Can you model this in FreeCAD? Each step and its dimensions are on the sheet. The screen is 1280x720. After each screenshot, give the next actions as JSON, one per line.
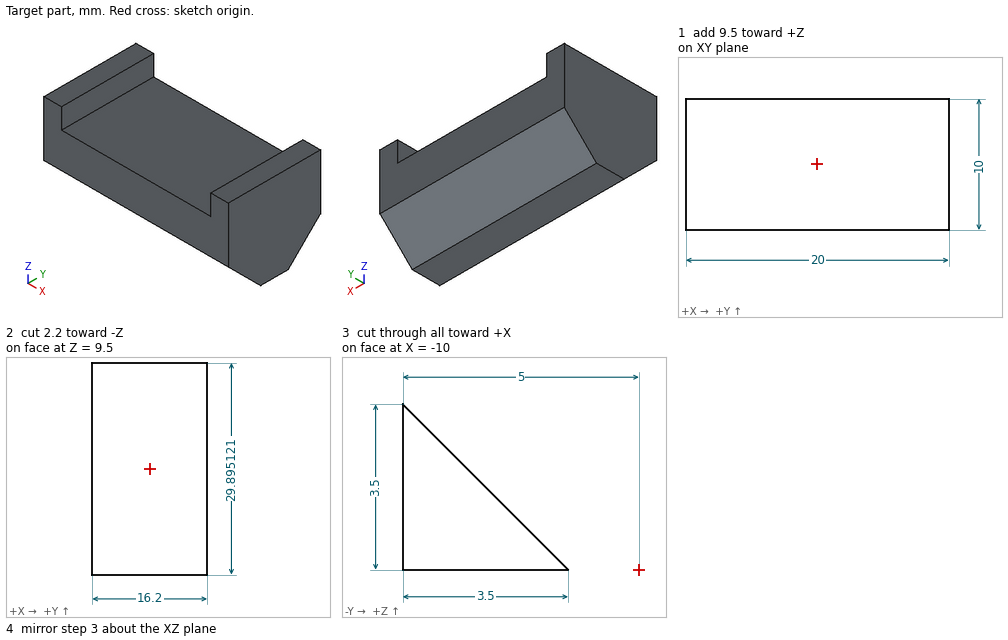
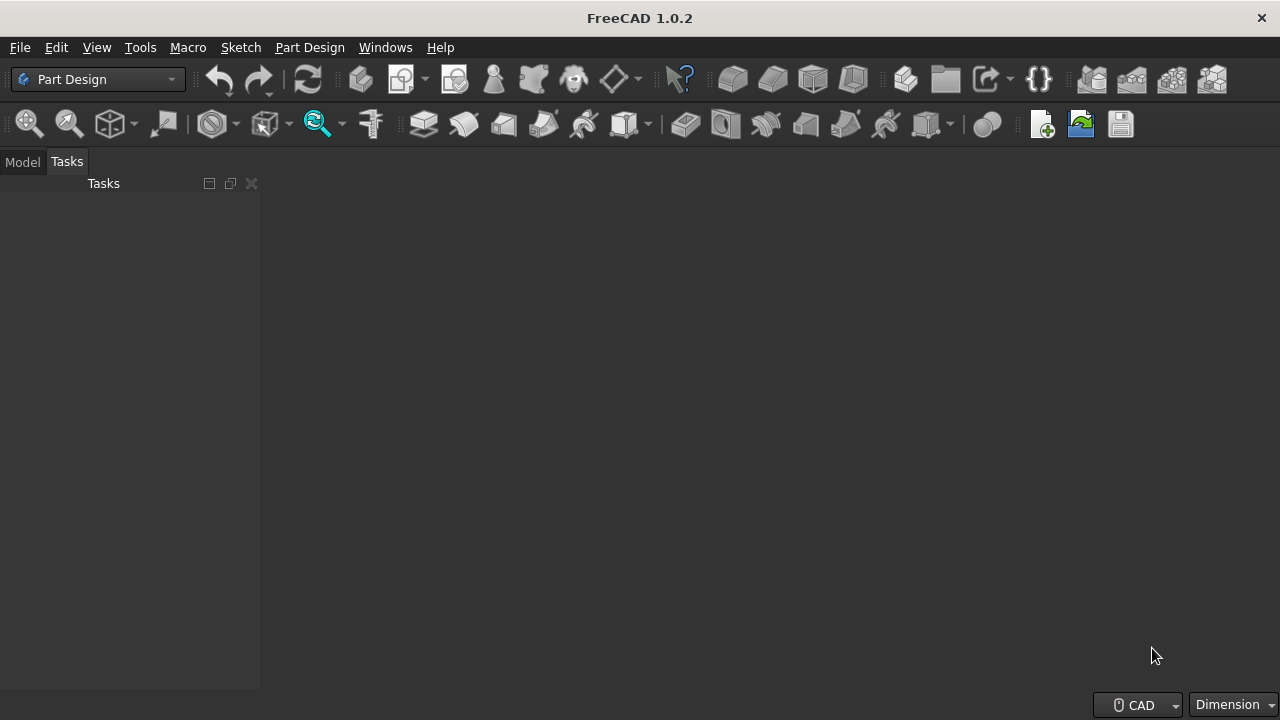
{"action": "left_click", "coordinate": [1042, 124]}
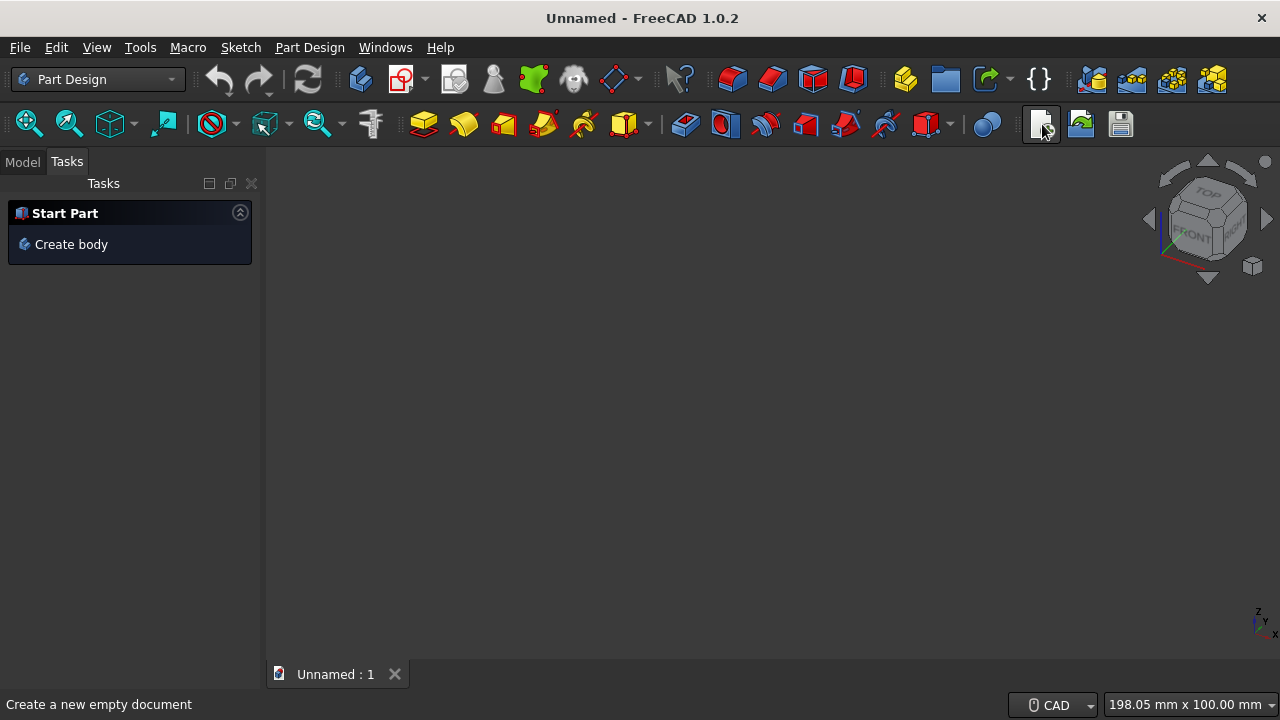
{"action": "left_click", "coordinate": [402, 80]}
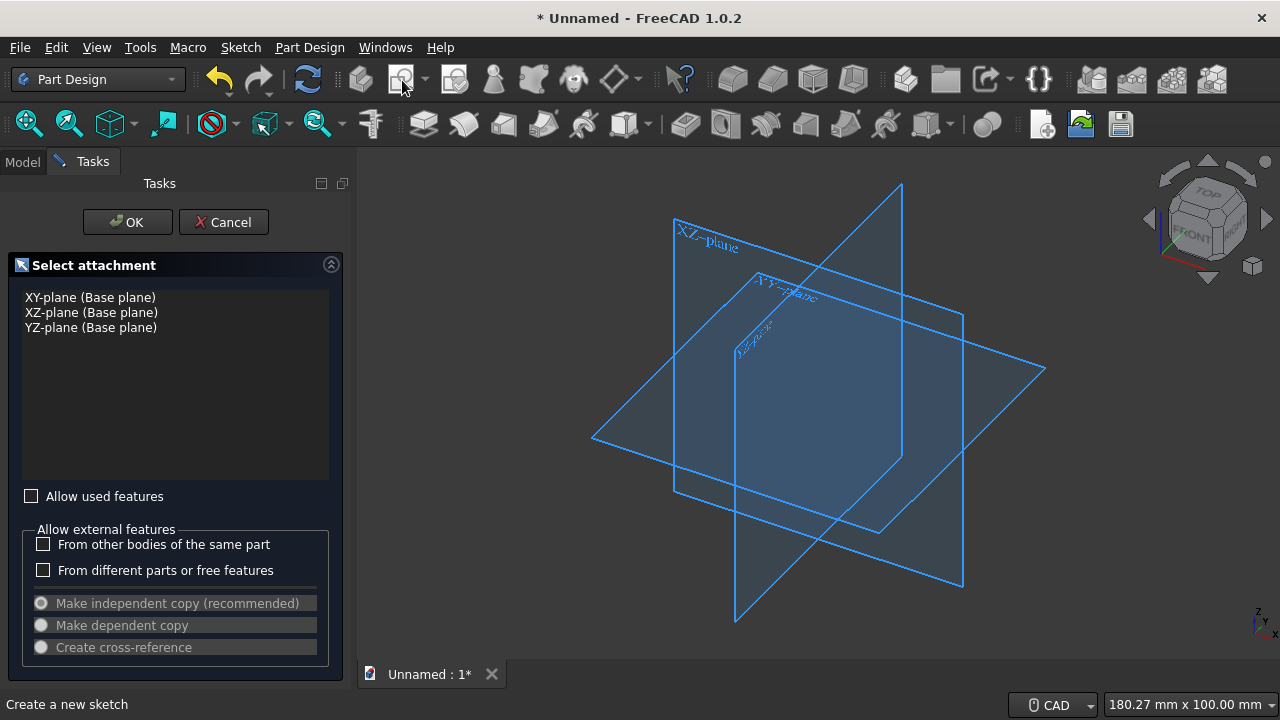
{"action": "left_click", "coordinate": [82, 298]}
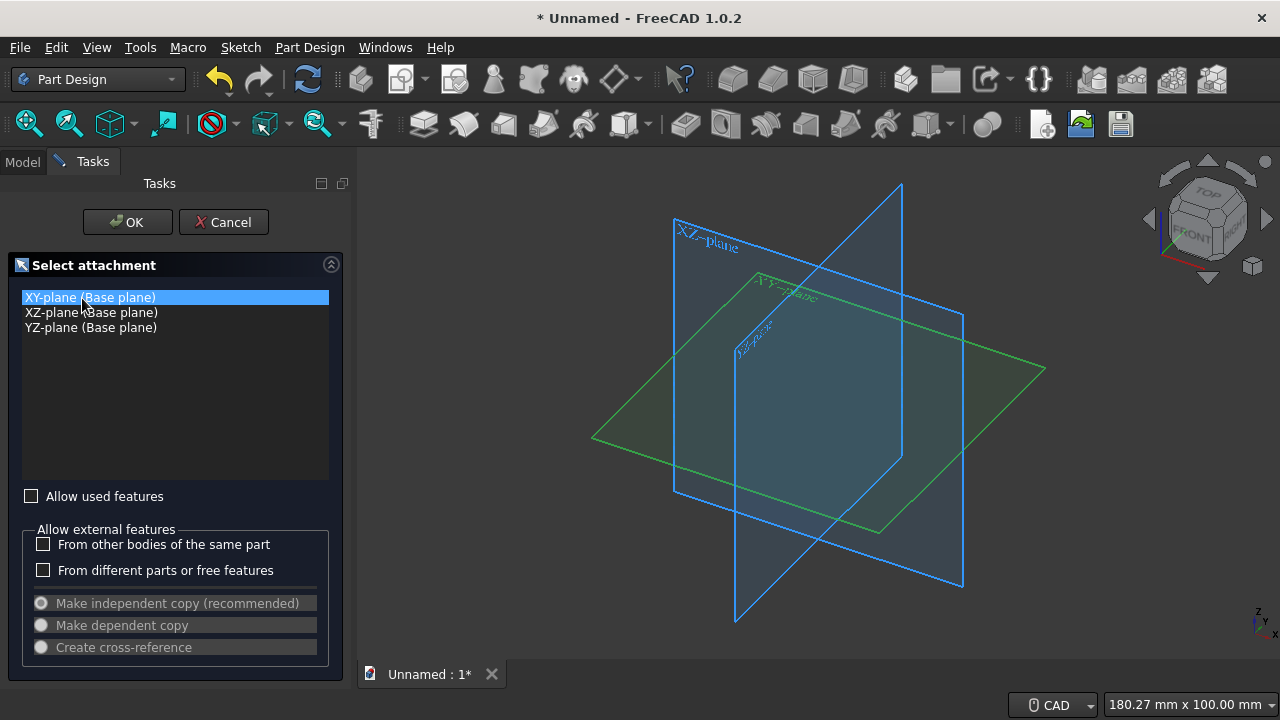
{"action": "left_click", "coordinate": [128, 222]}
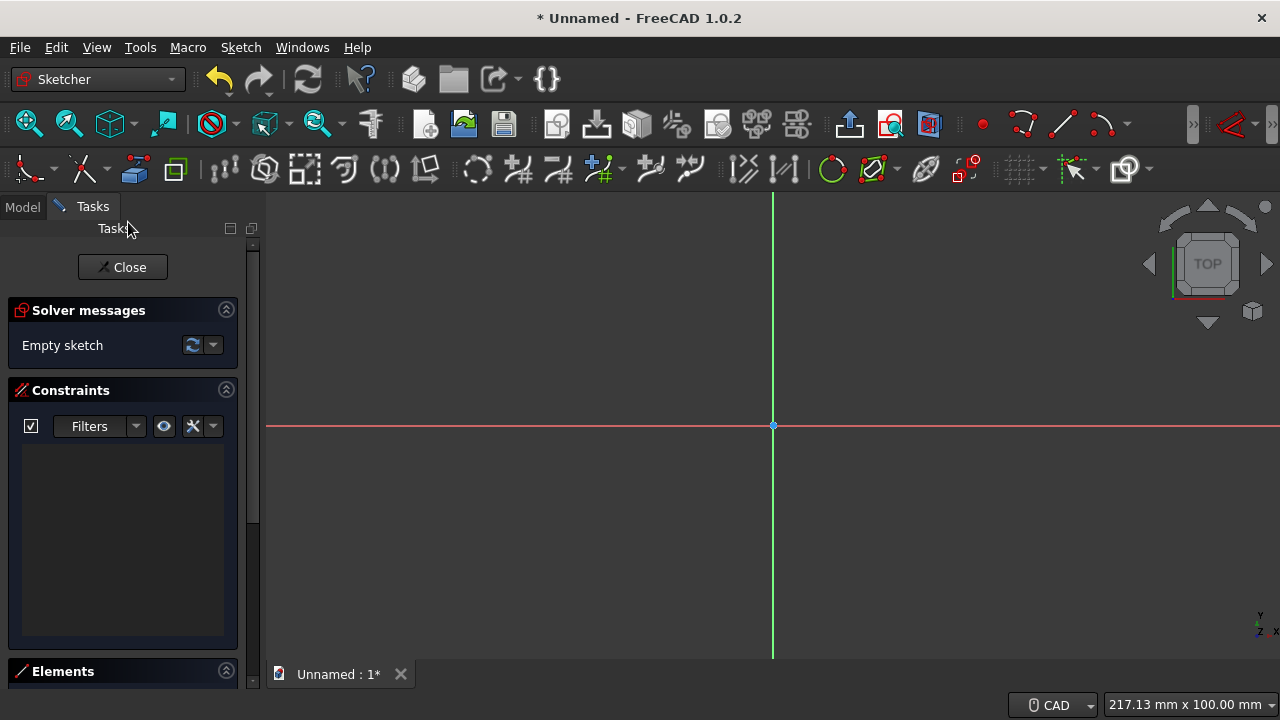
{"action": "scroll", "coordinate": [787, 426], "scroll_direction": "up", "scroll_amount": 9}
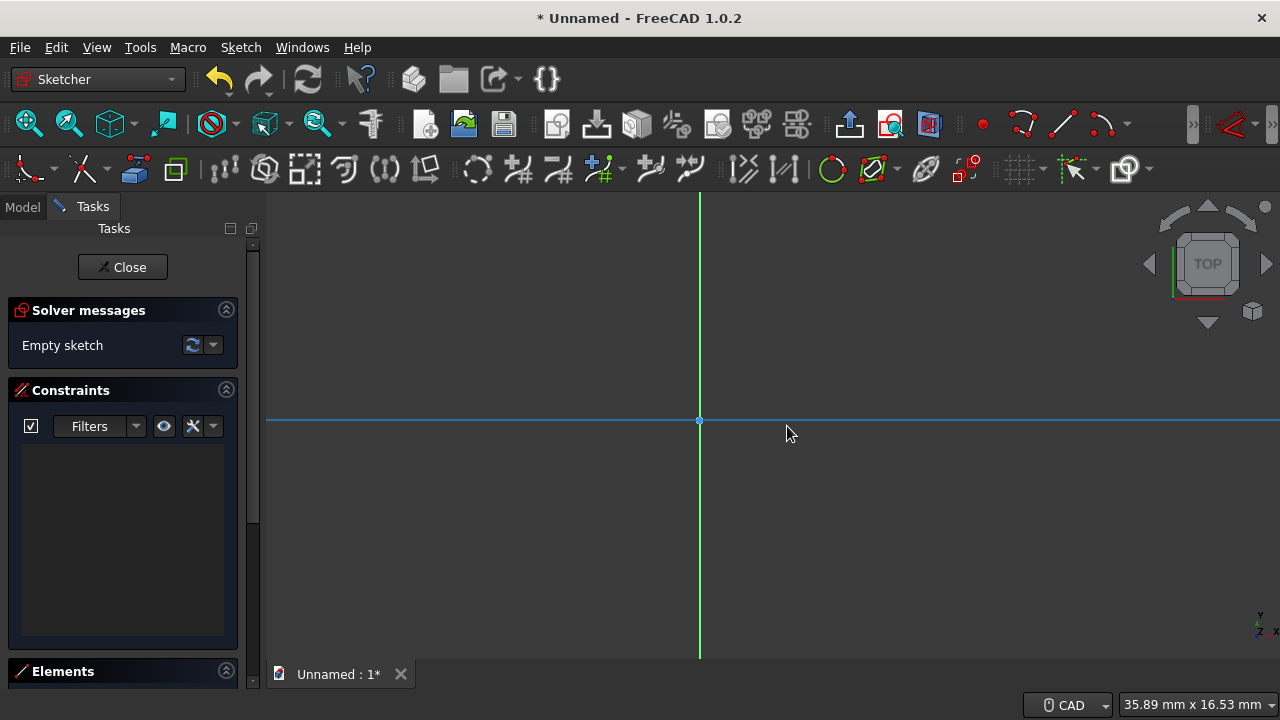
{"action": "key", "text": "g v"}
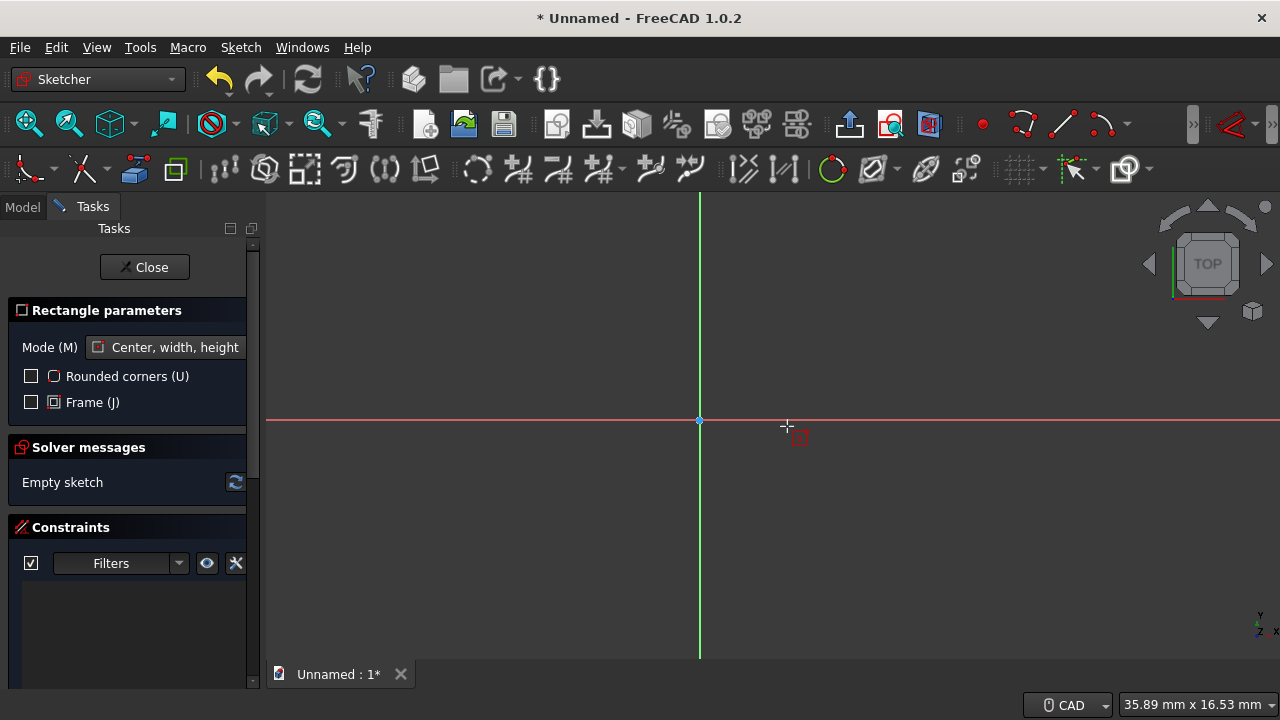
{"action": "left_click", "coordinate": [700, 420]}
{"action": "left_click", "coordinate": [982, 279]}
{"action": "key", "text": "Escape"}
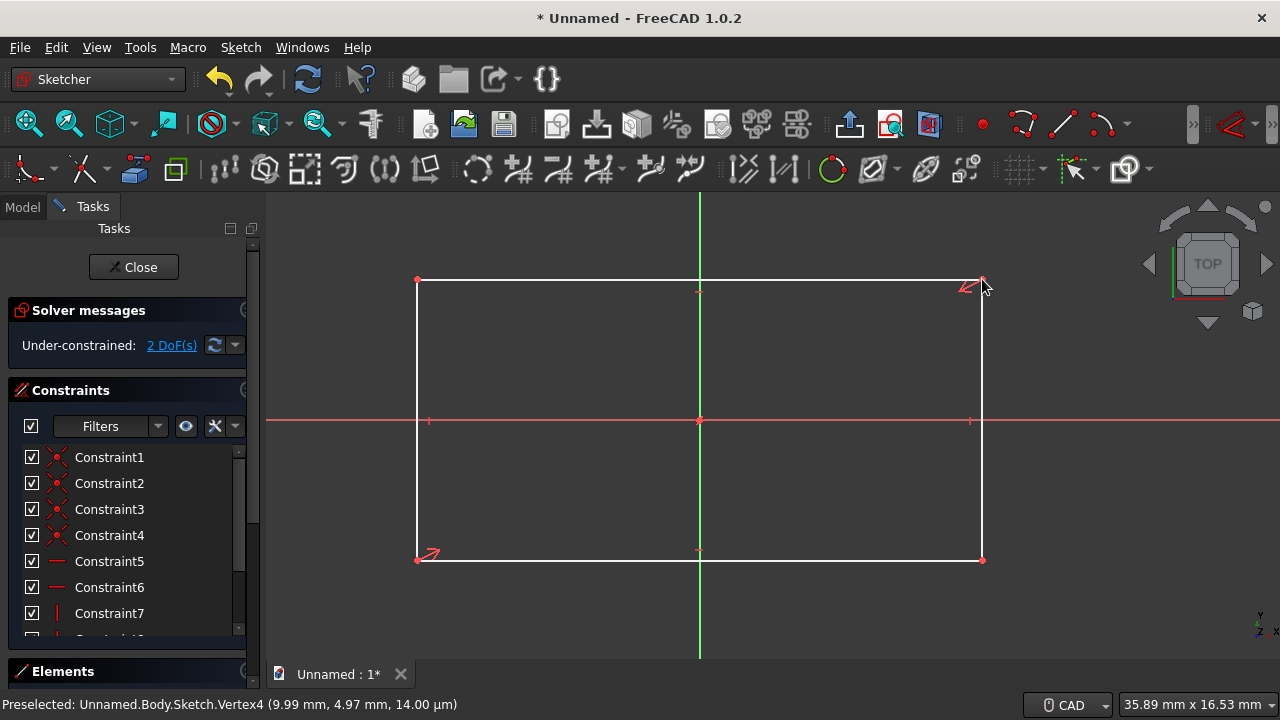
{"action": "left_click", "coordinate": [587, 561]}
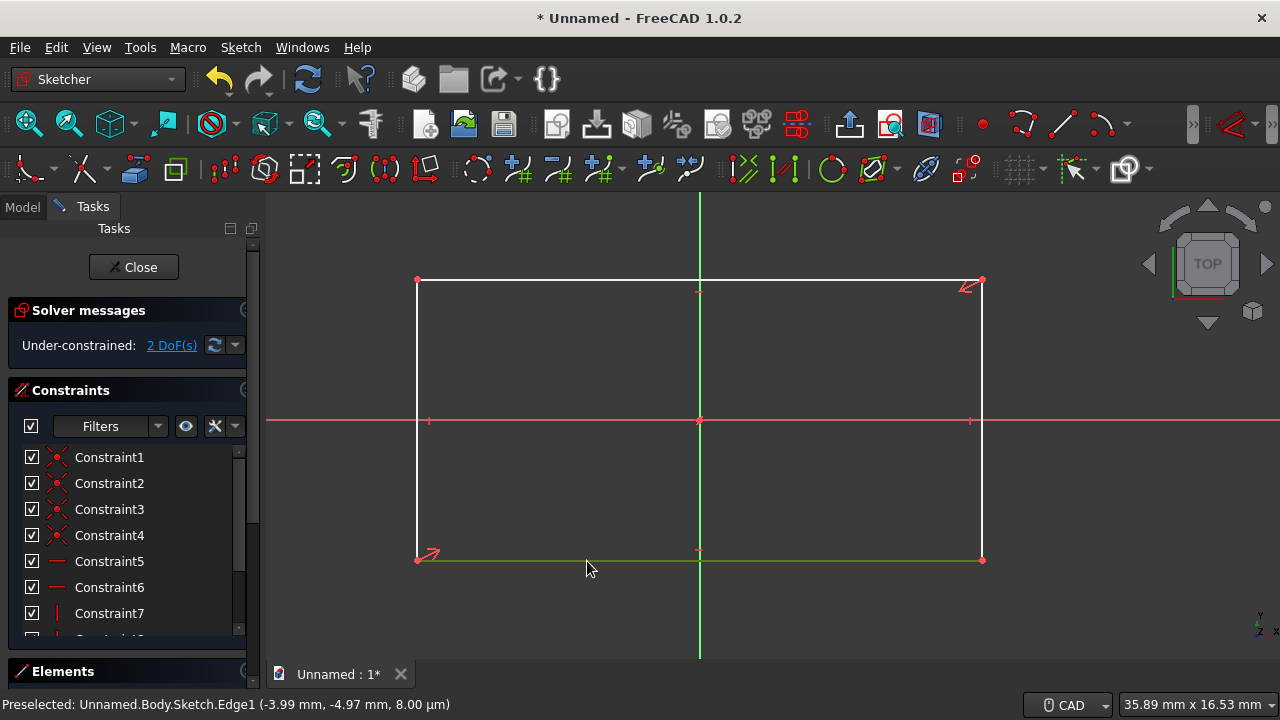
{"action": "left_click", "coordinate": [1258, 124]}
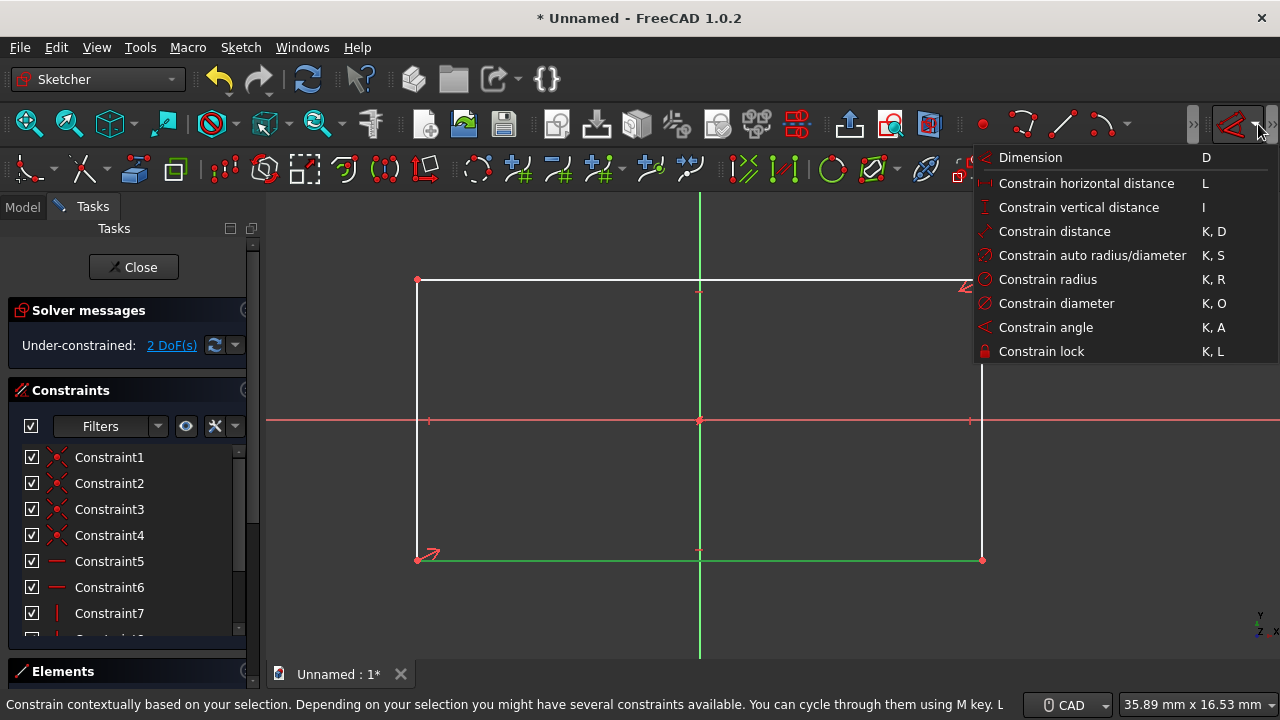
{"action": "left_click", "coordinate": [1126, 183]}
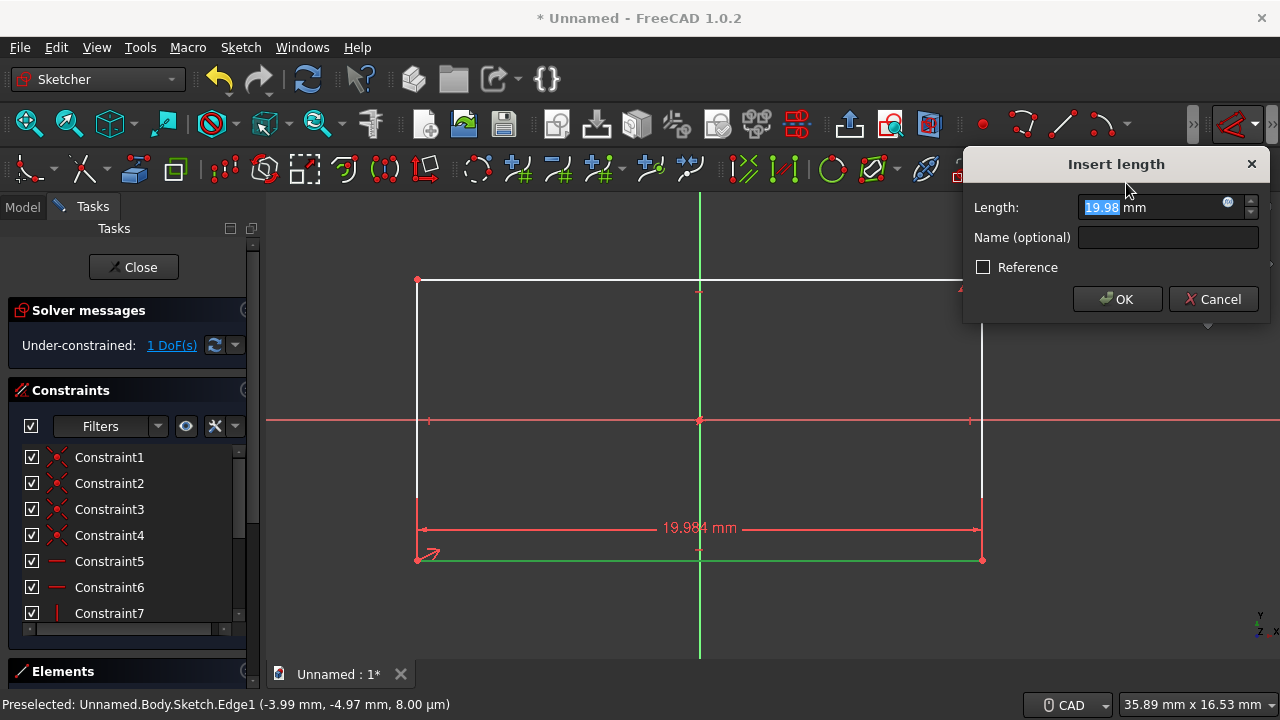
{"action": "type", "text": "20"}
{"action": "key", "text": "Return"}